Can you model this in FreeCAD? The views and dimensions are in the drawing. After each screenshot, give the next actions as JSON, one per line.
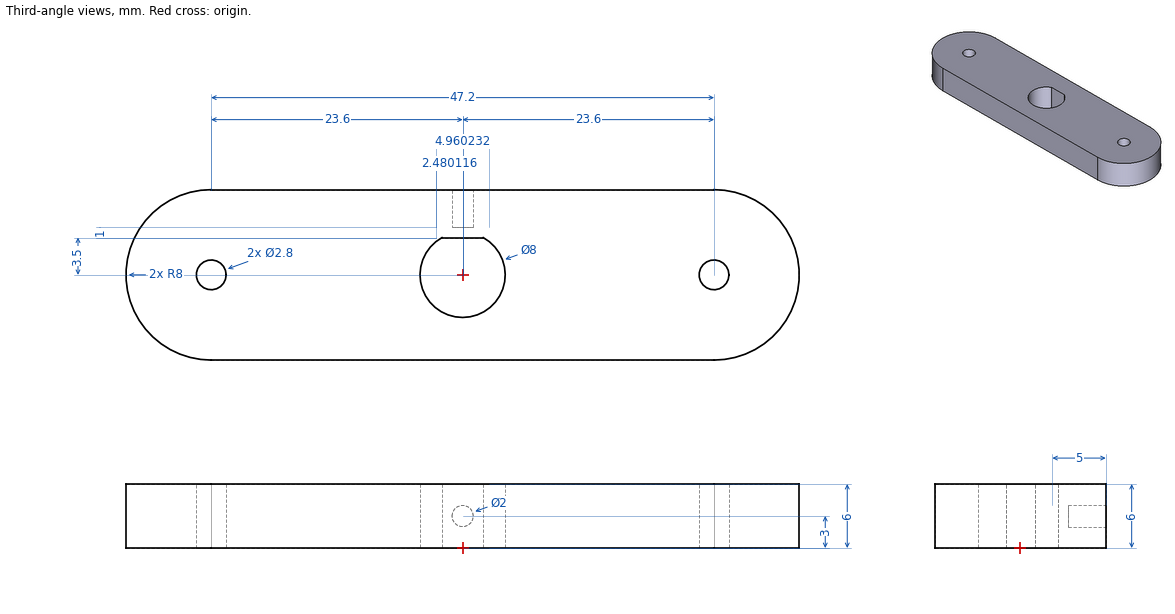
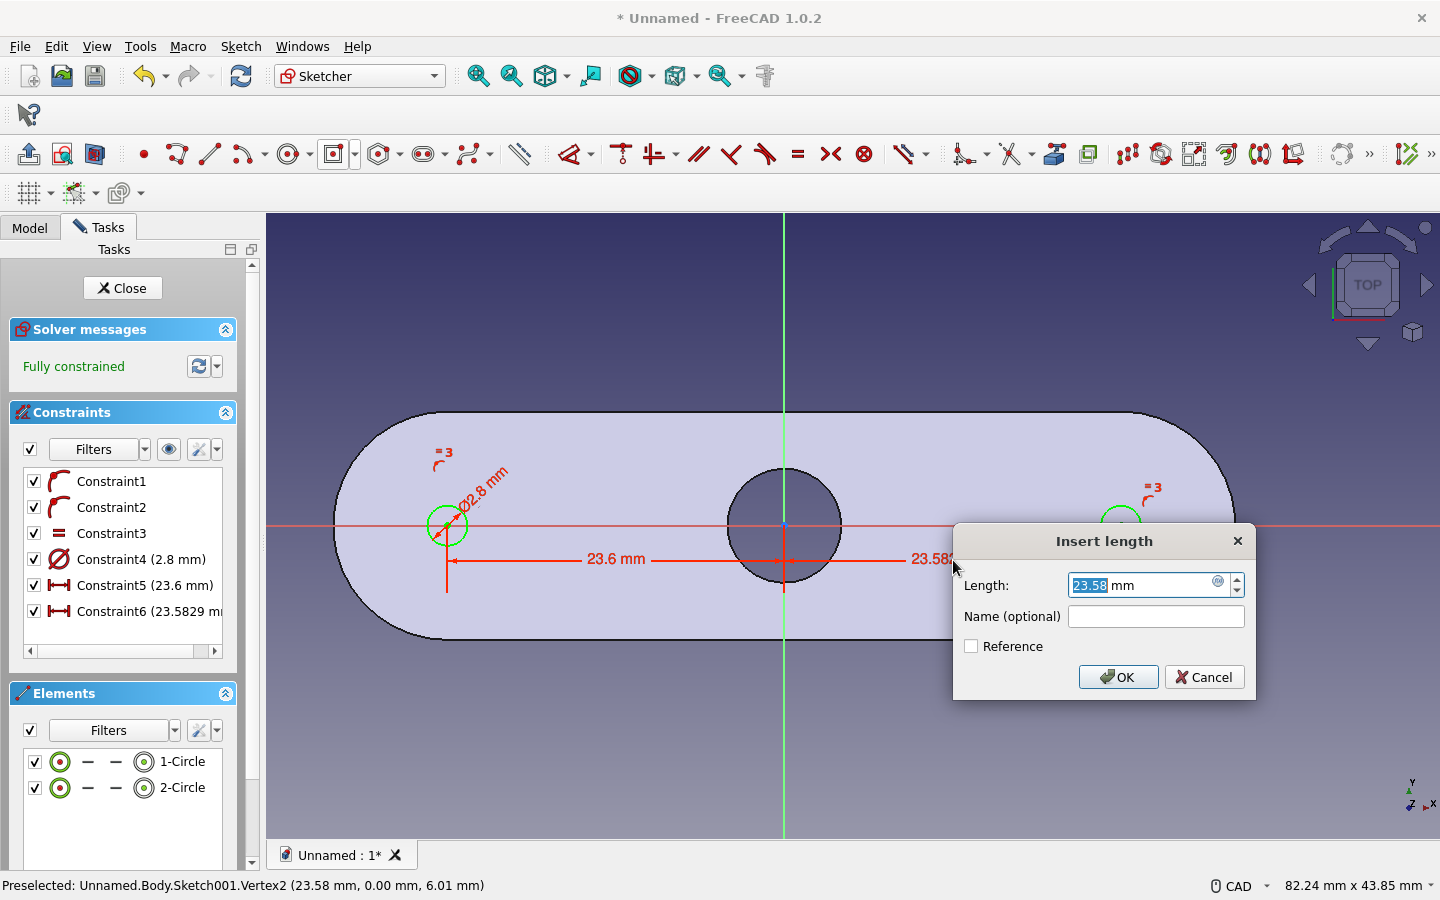
{"action": "type", "text": "23.6"}
{"action": "key", "text": "Return"}
{"action": "key", "text": "Escape"}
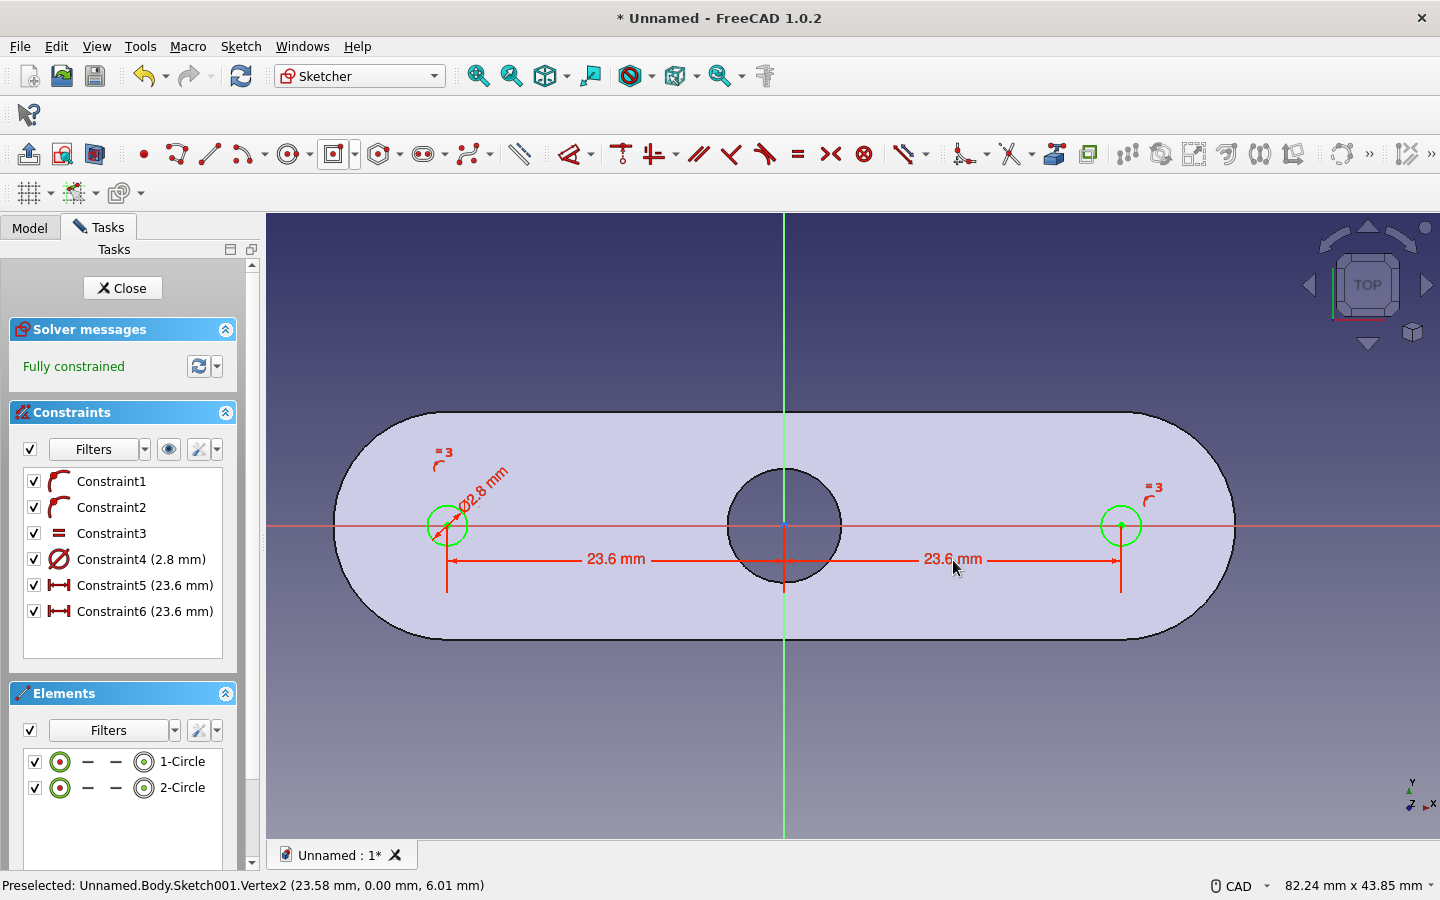
{"action": "left_click", "coordinate": [123, 288]}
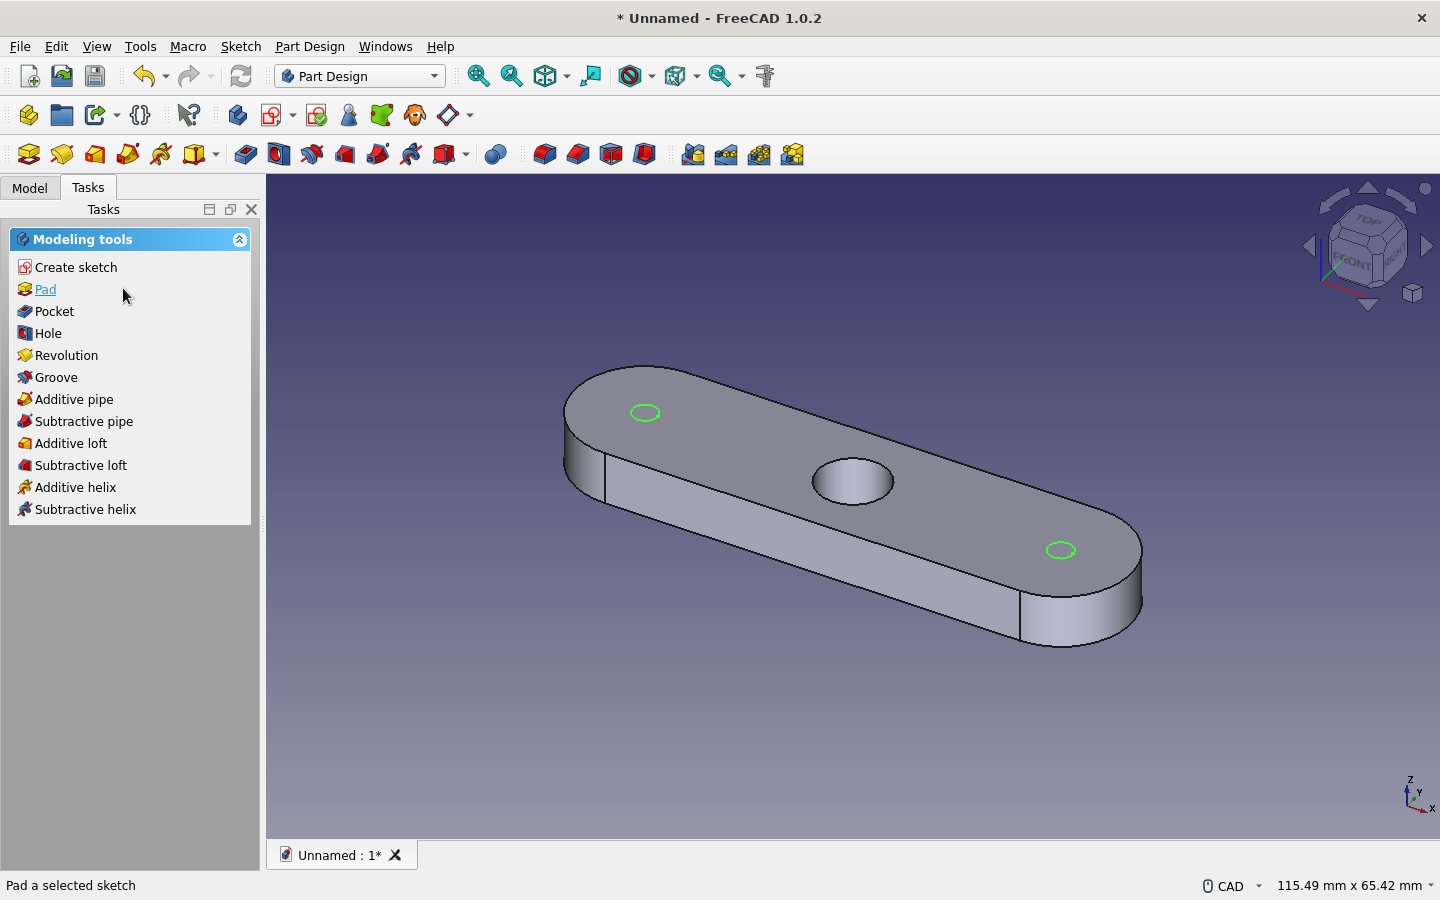
{"action": "left_click", "coordinate": [246, 154]}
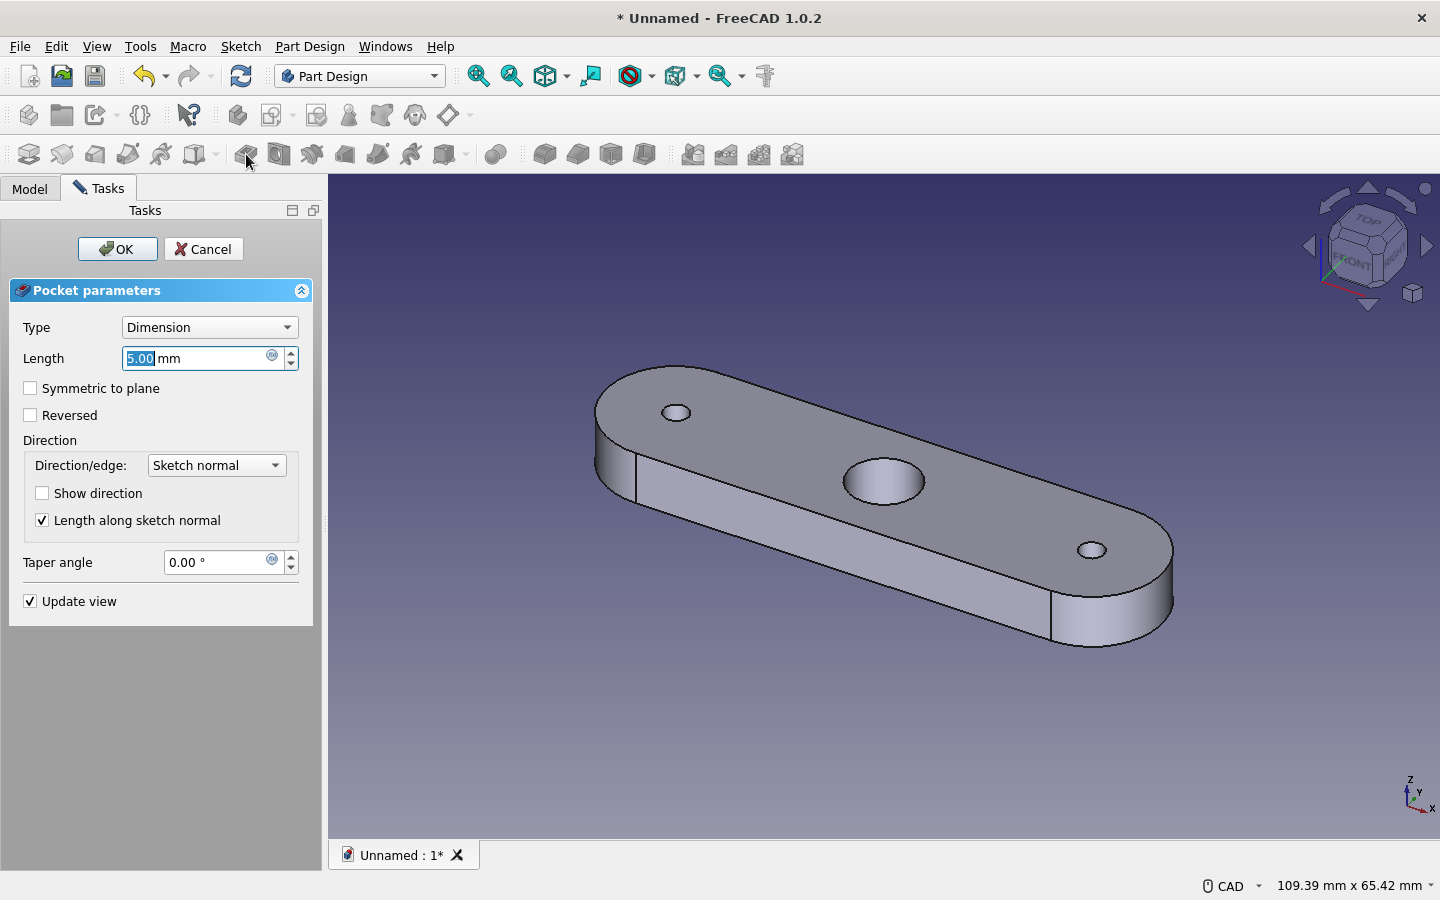
{"action": "left_click", "coordinate": [210, 328]}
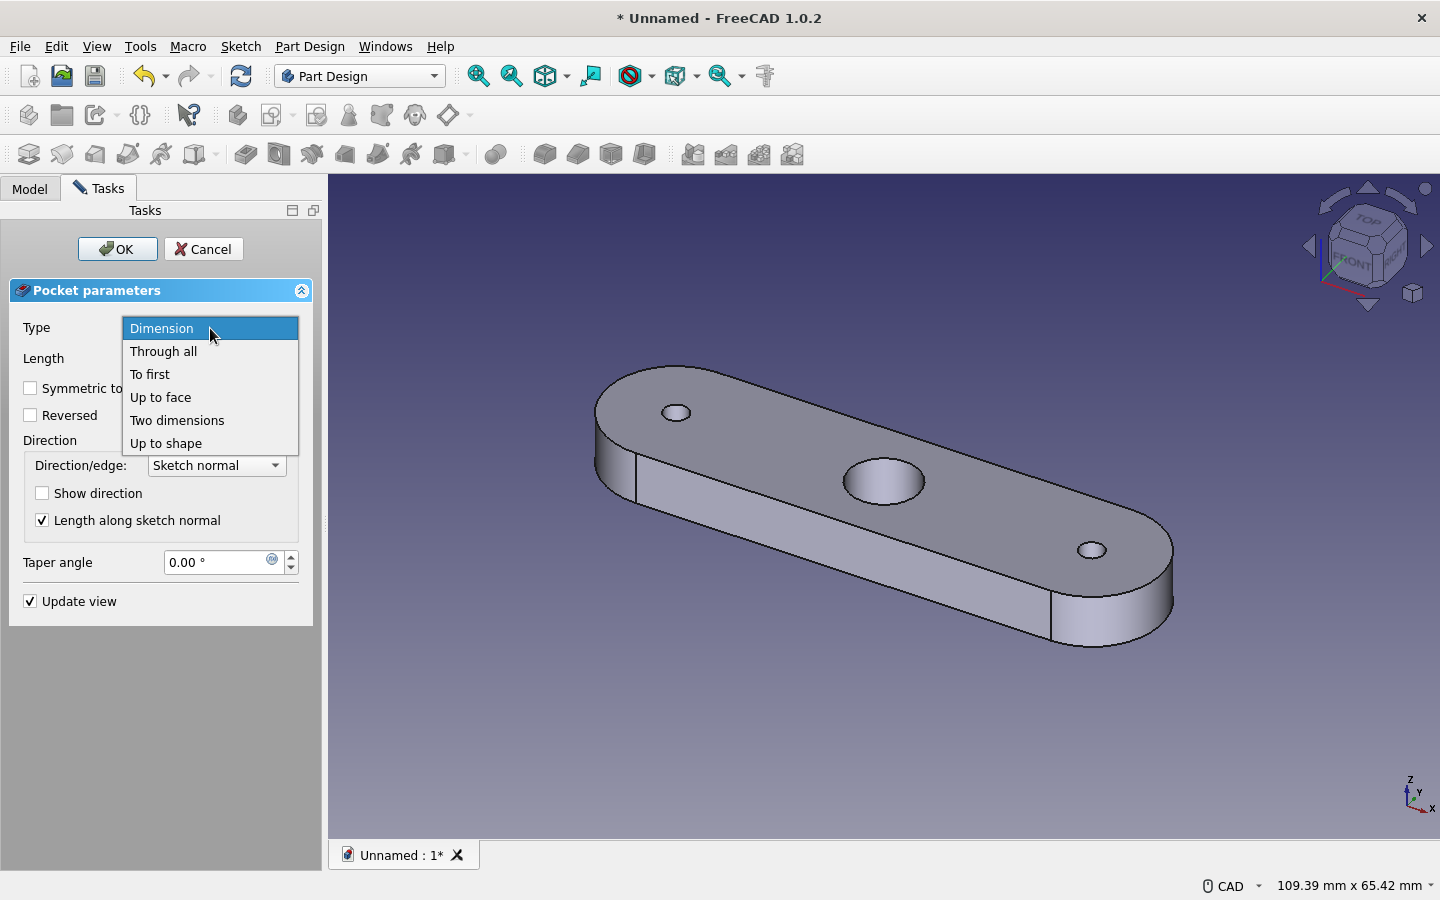
{"action": "left_click", "coordinate": [208, 352]}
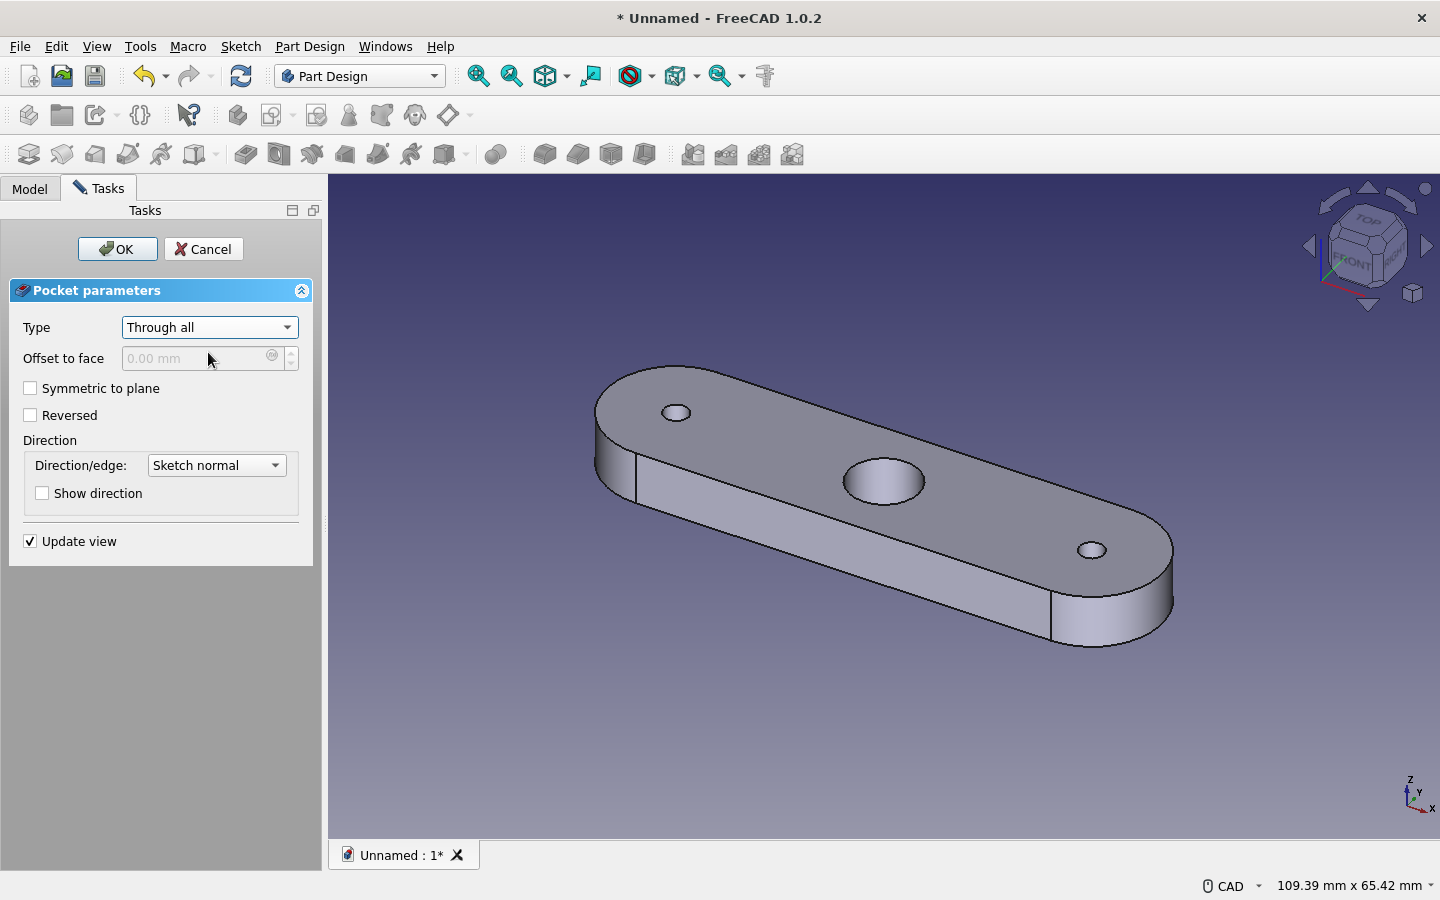
{"action": "left_click", "coordinate": [118, 249]}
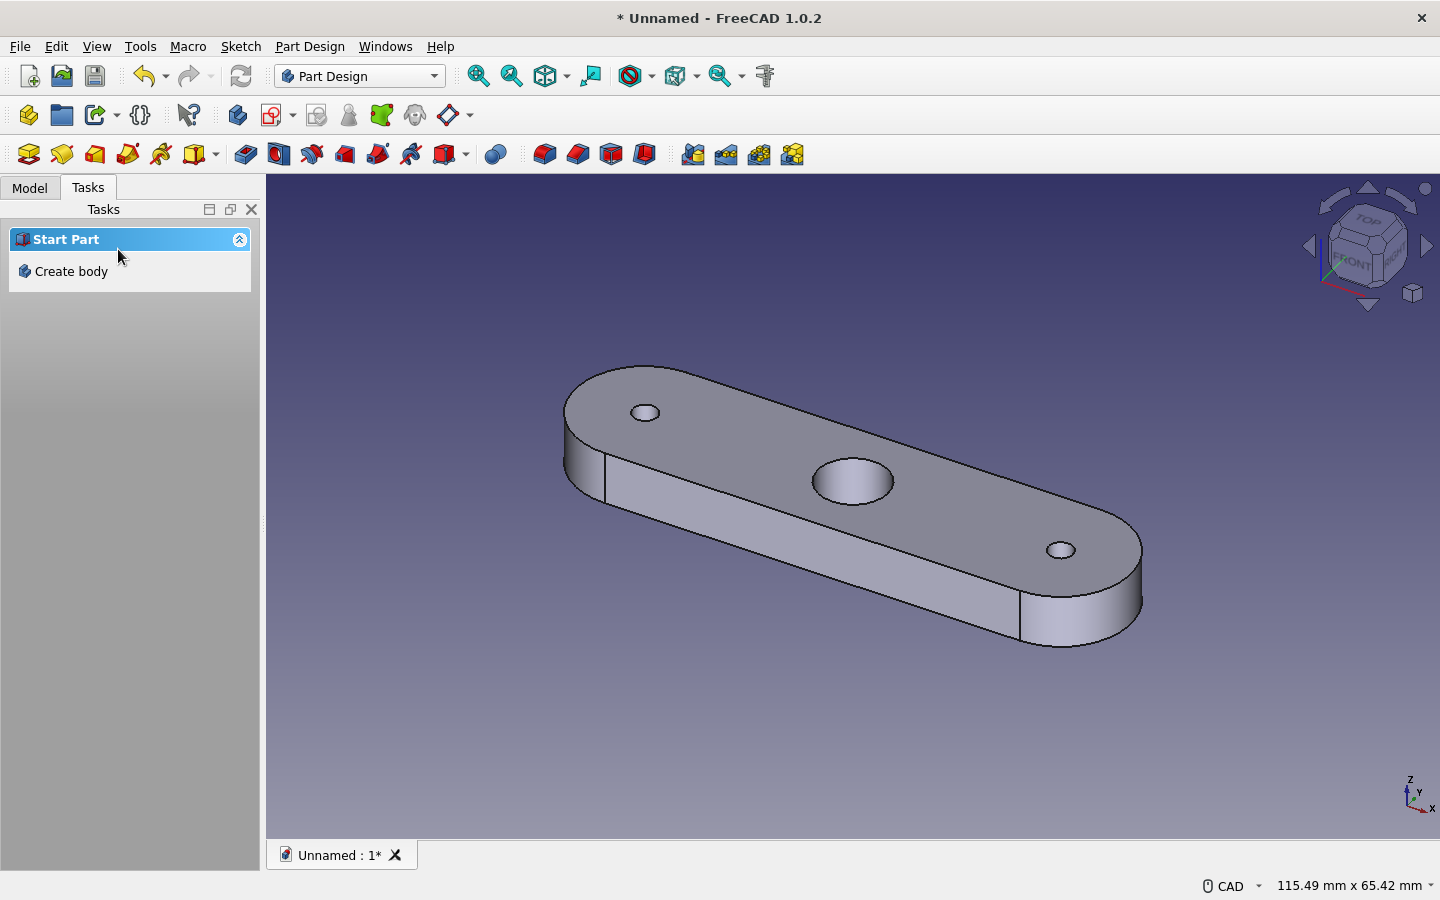
{"action": "key", "text": "4"}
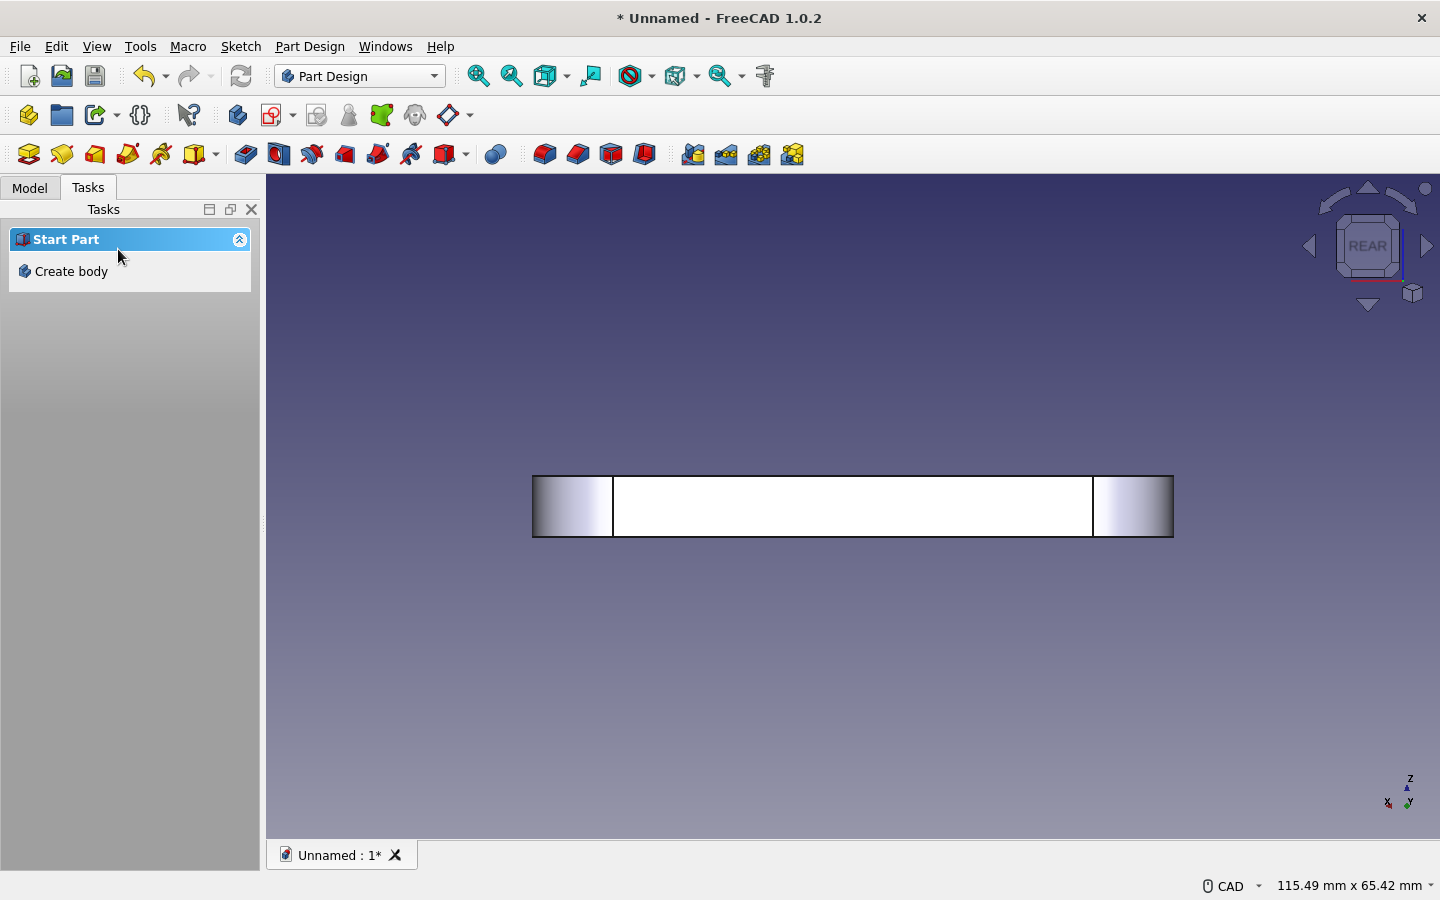
{"action": "left_click", "coordinate": [647, 505]}